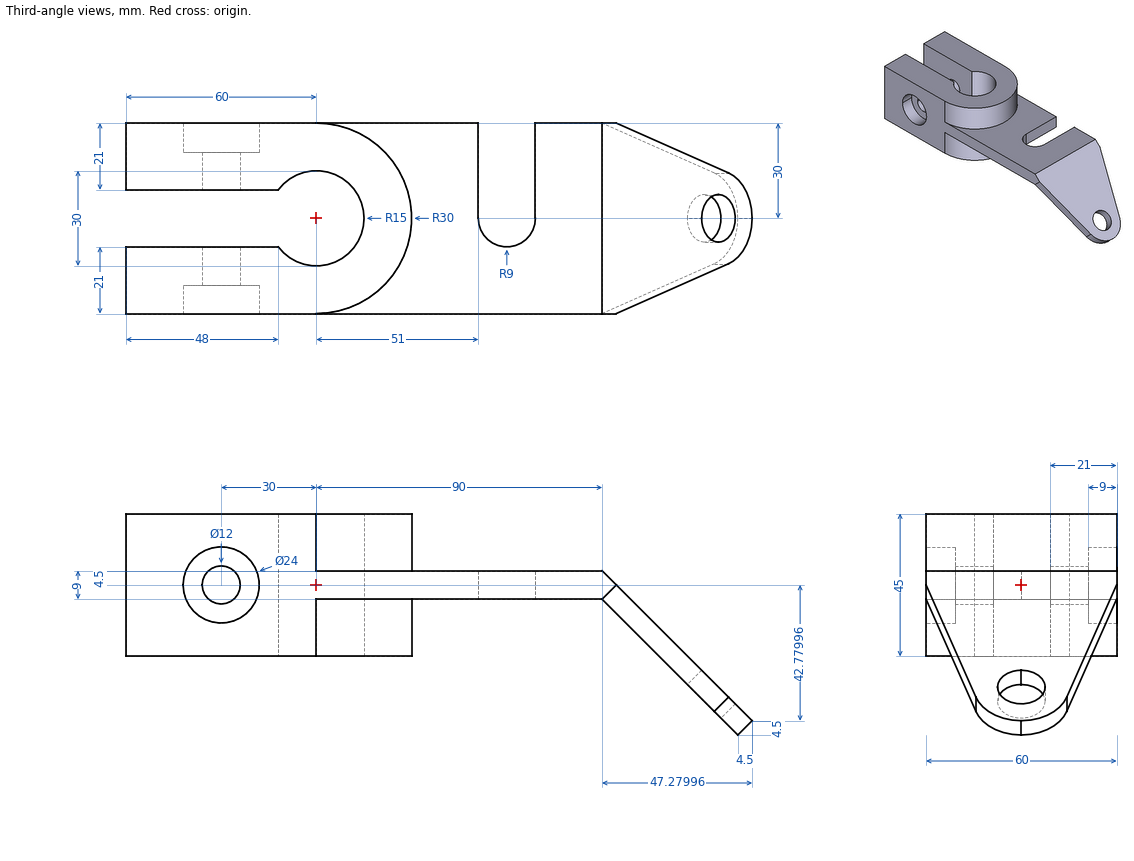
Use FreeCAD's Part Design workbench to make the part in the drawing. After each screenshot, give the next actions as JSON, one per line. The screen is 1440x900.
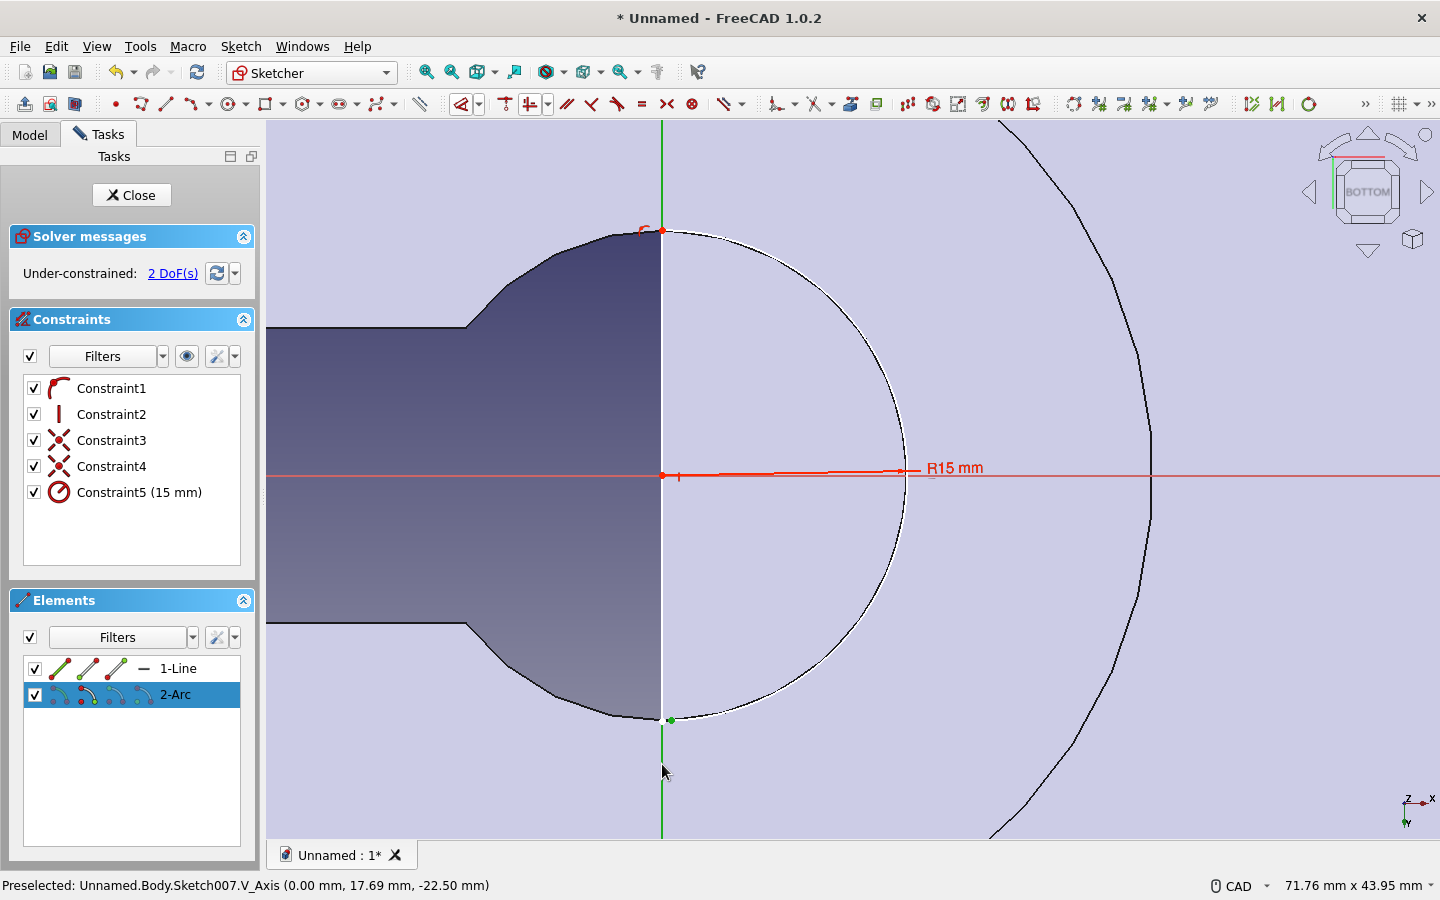
{"action": "left_click", "coordinate": [505, 104]}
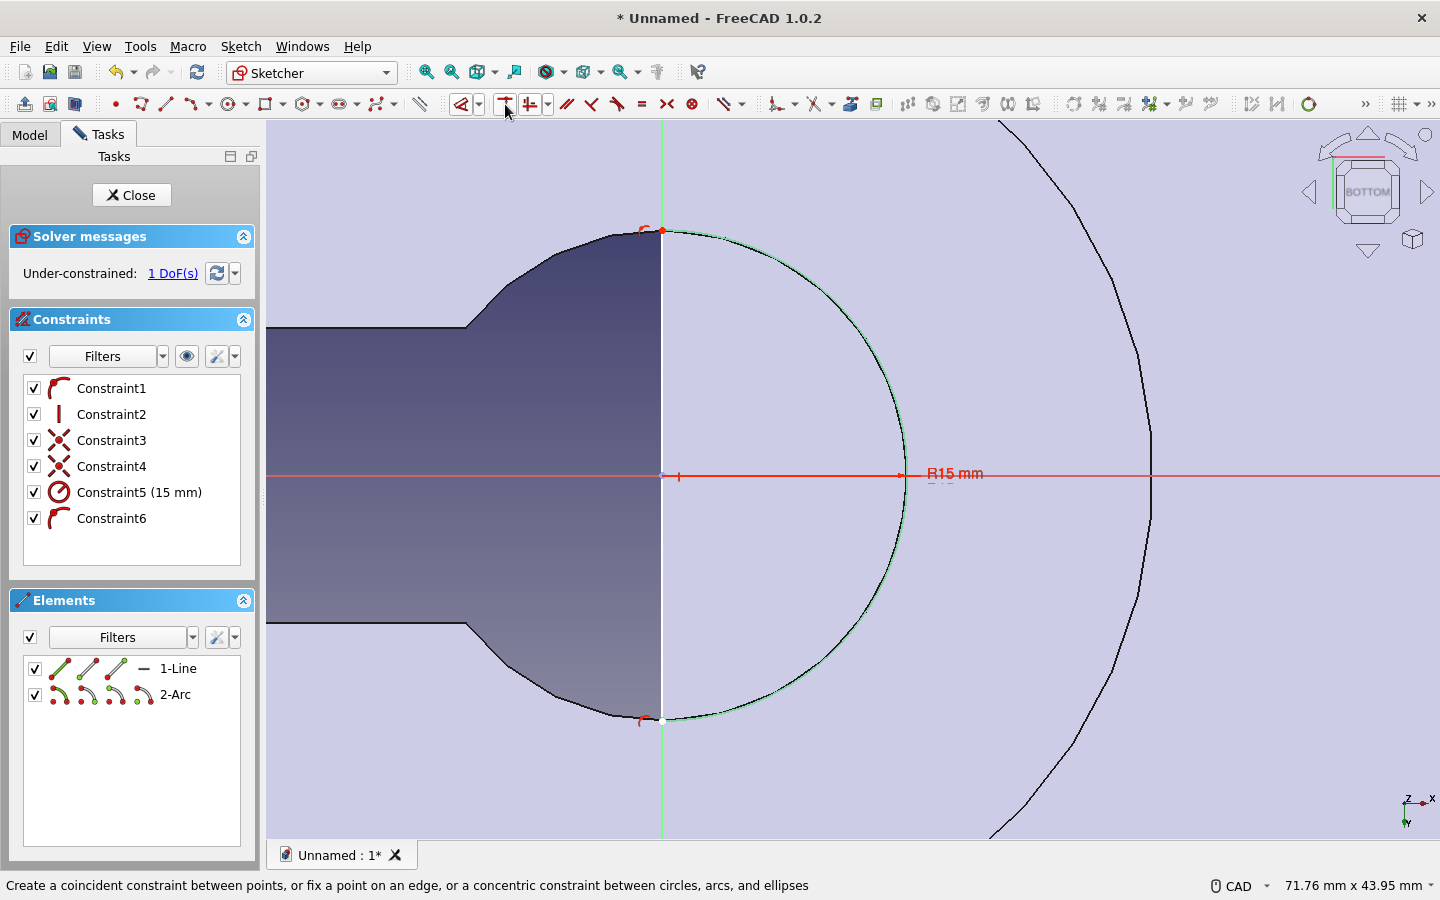
{"action": "left_click", "coordinate": [662, 378]}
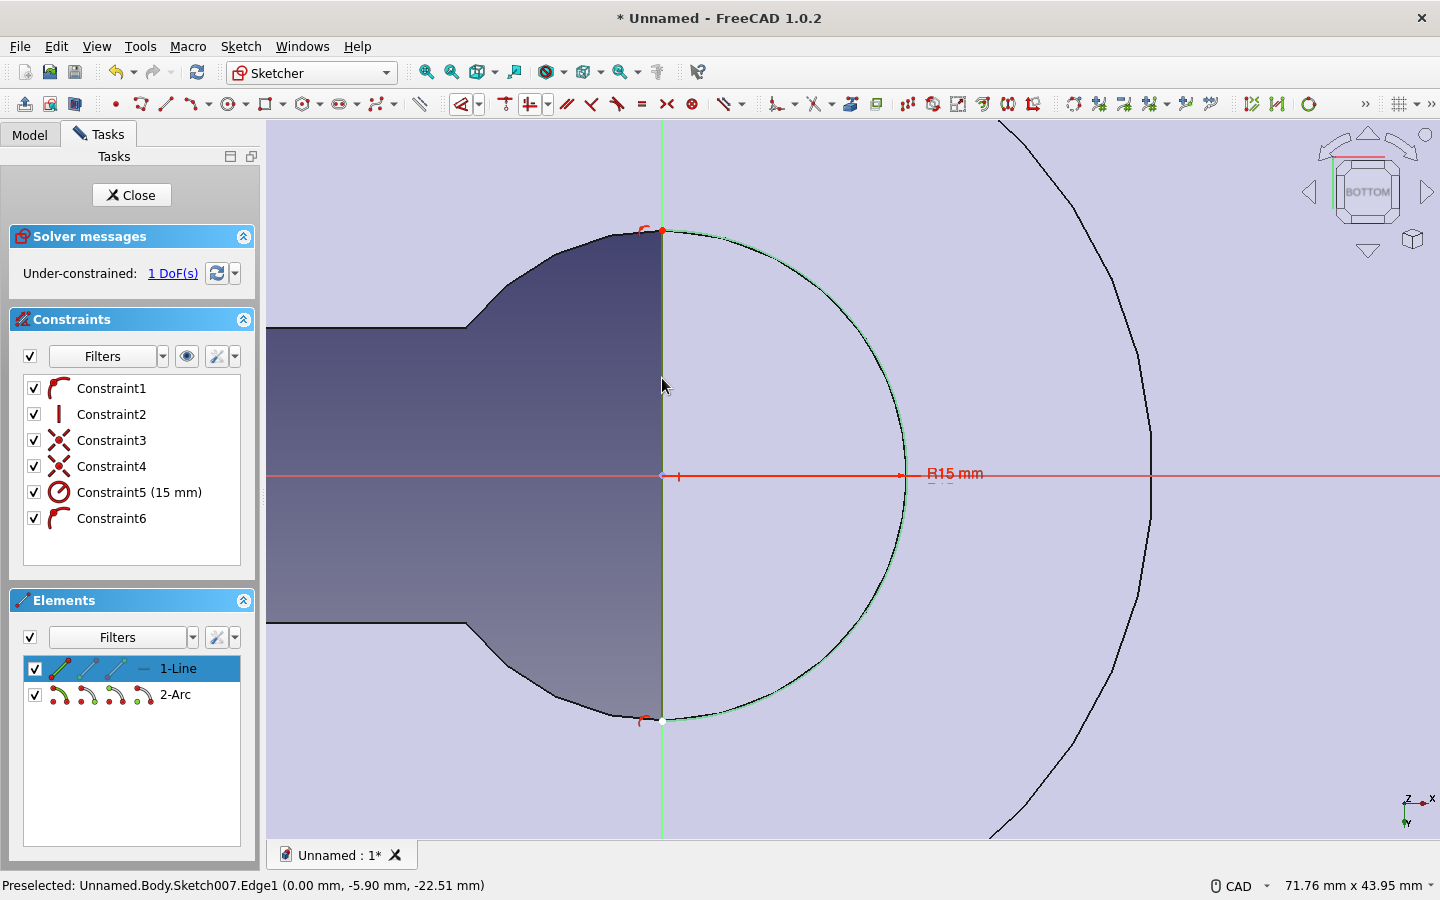
{"action": "left_click", "coordinate": [478, 104]}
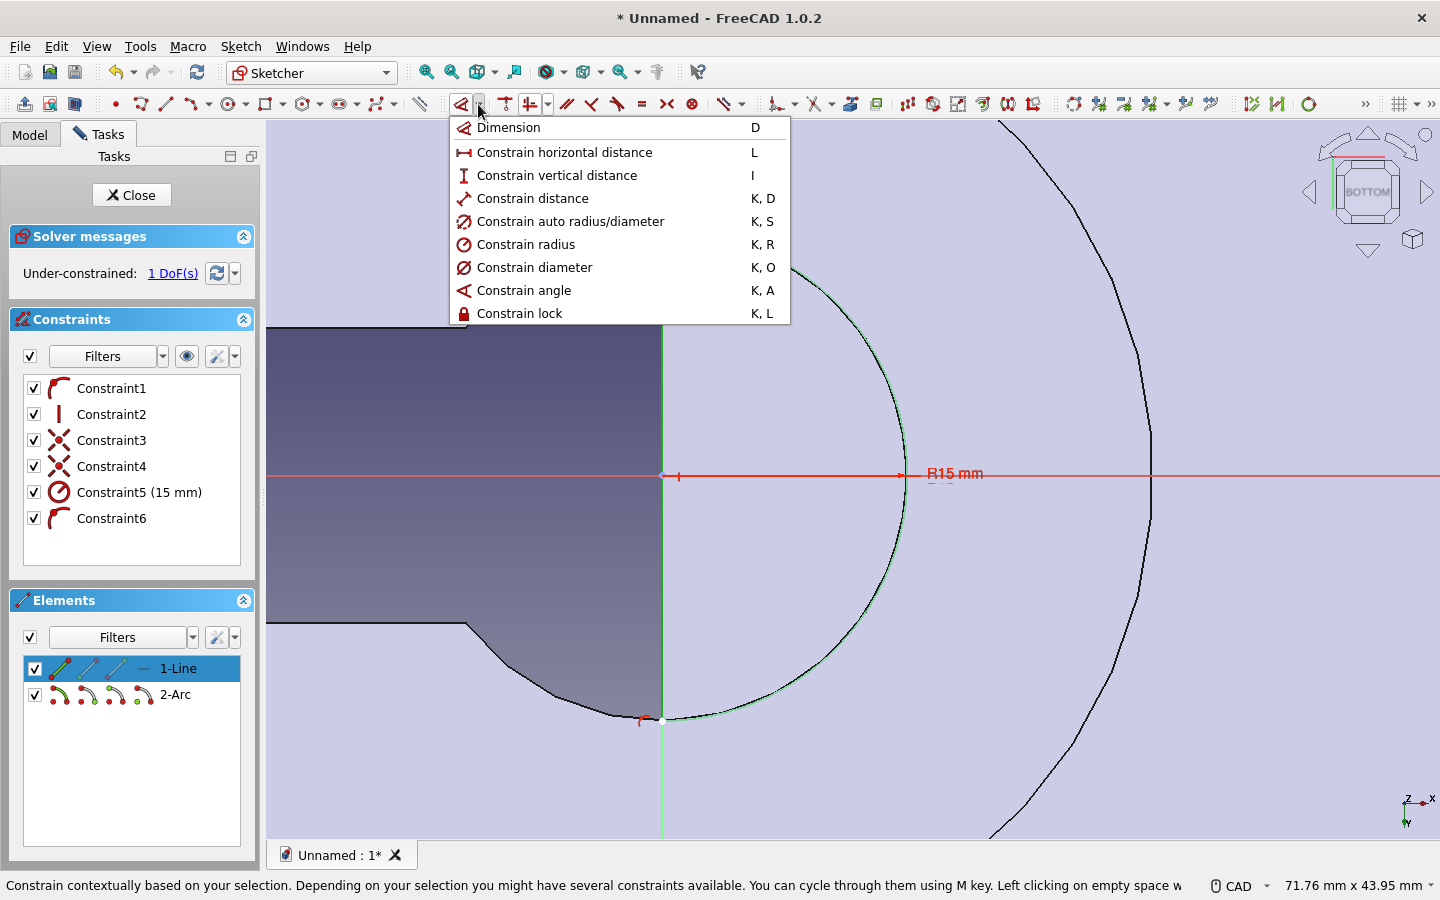
{"action": "left_click", "coordinate": [620, 176]}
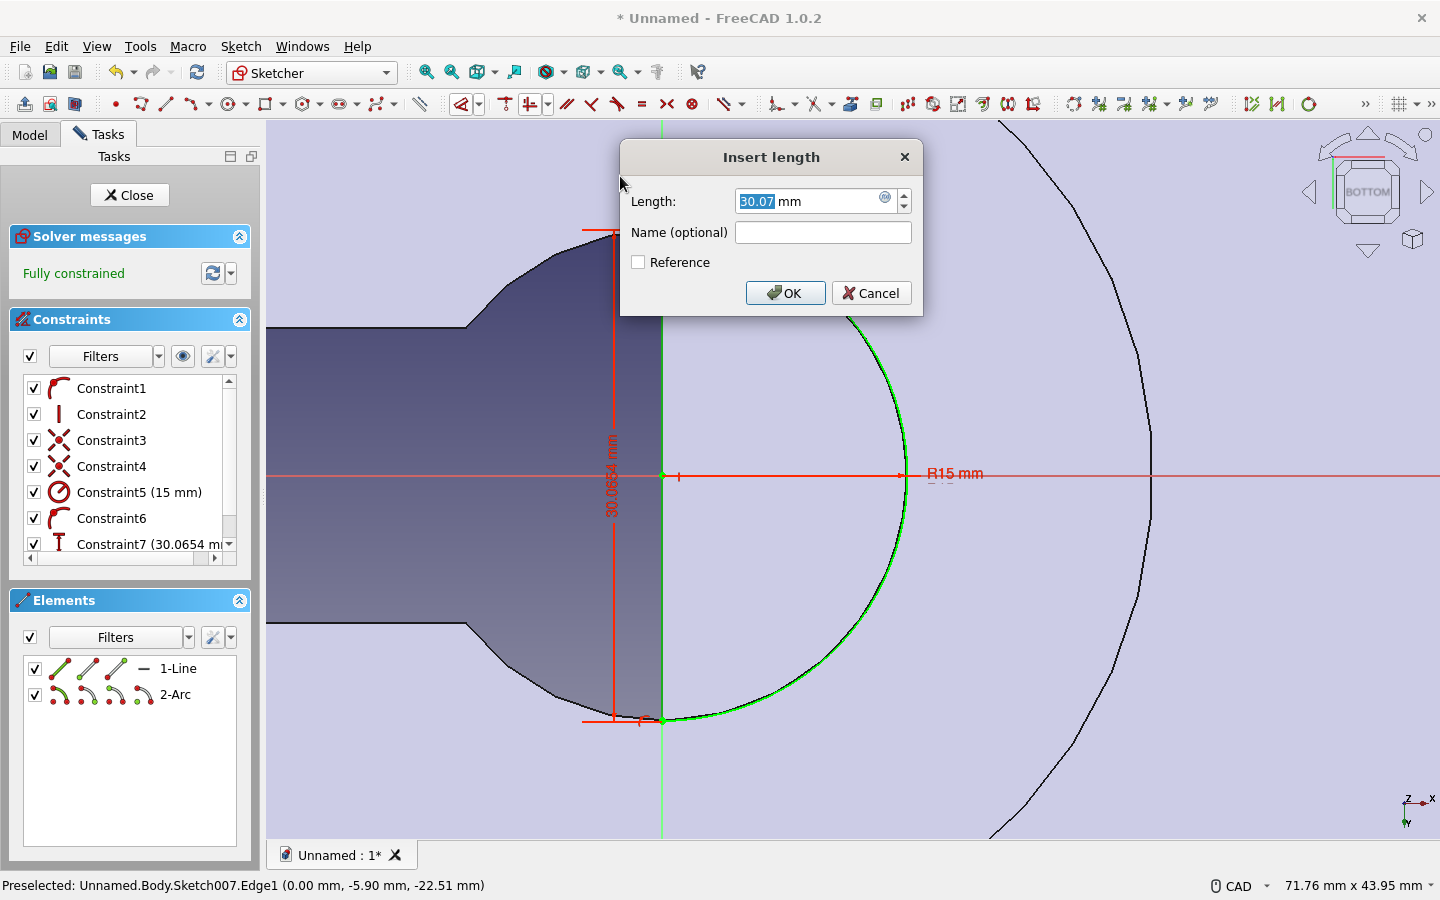
{"action": "type", "text": "30"}
{"action": "key", "text": "Return"}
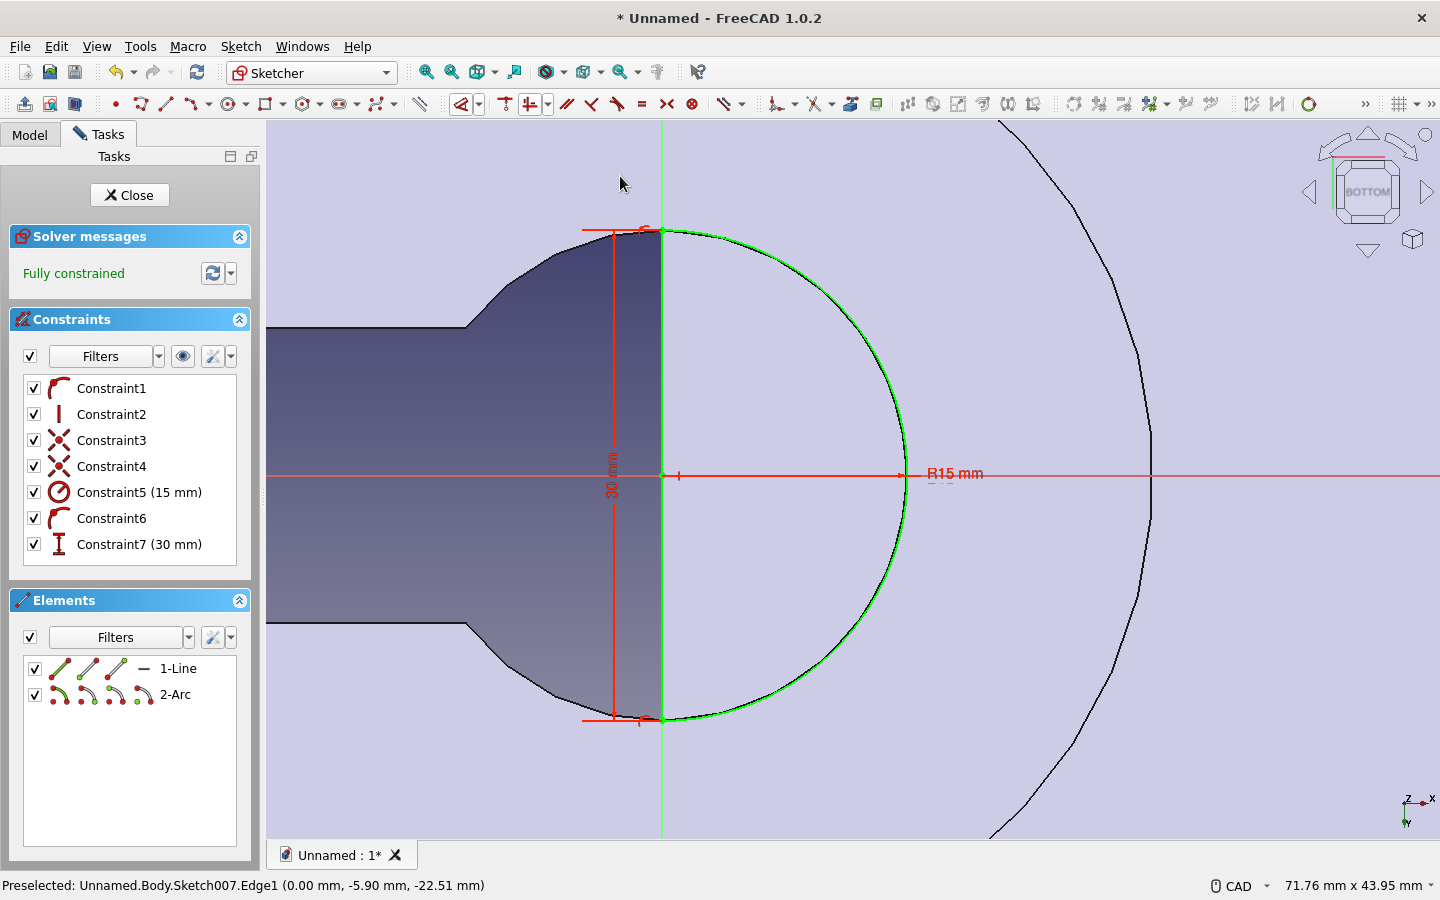
{"action": "left_click", "coordinate": [130, 195]}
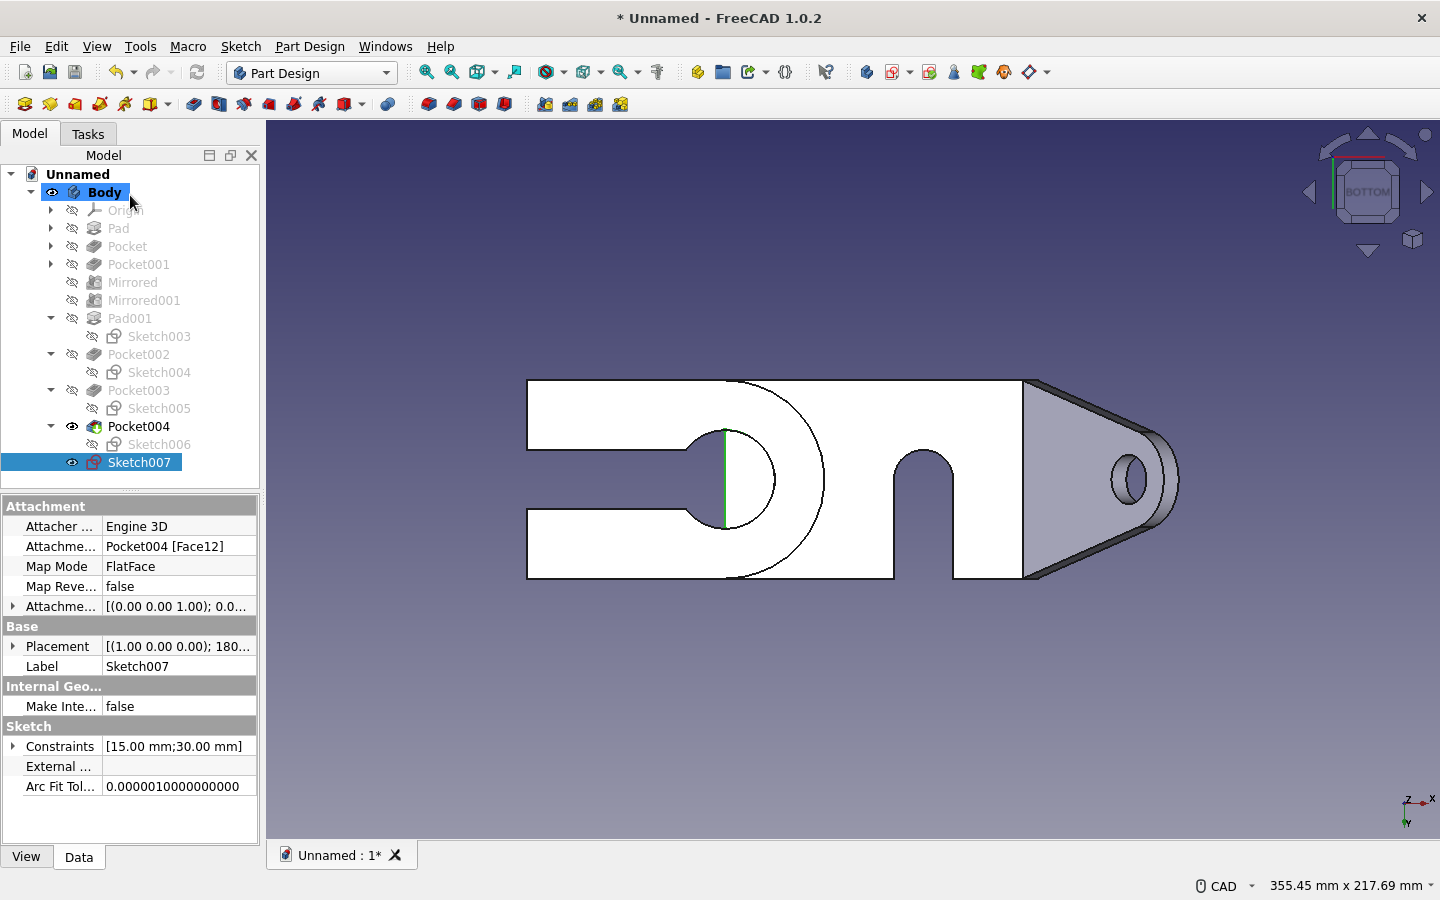
{"action": "left_click", "coordinate": [194, 104]}